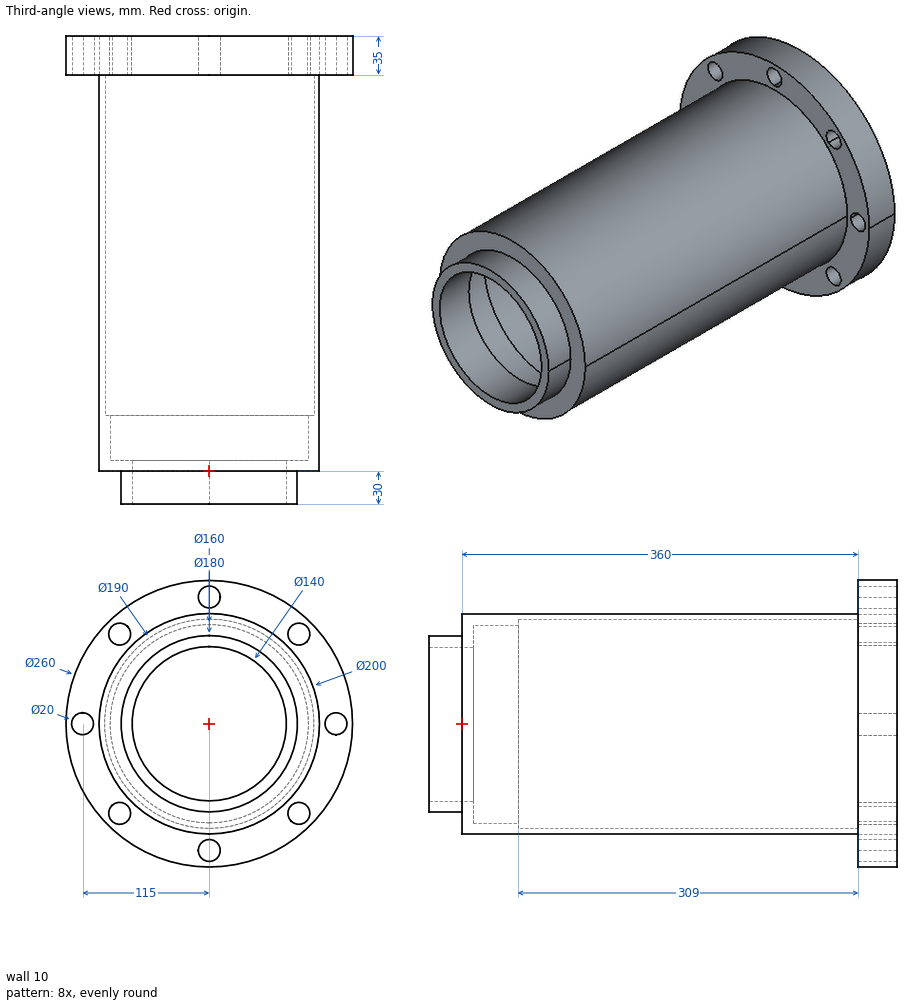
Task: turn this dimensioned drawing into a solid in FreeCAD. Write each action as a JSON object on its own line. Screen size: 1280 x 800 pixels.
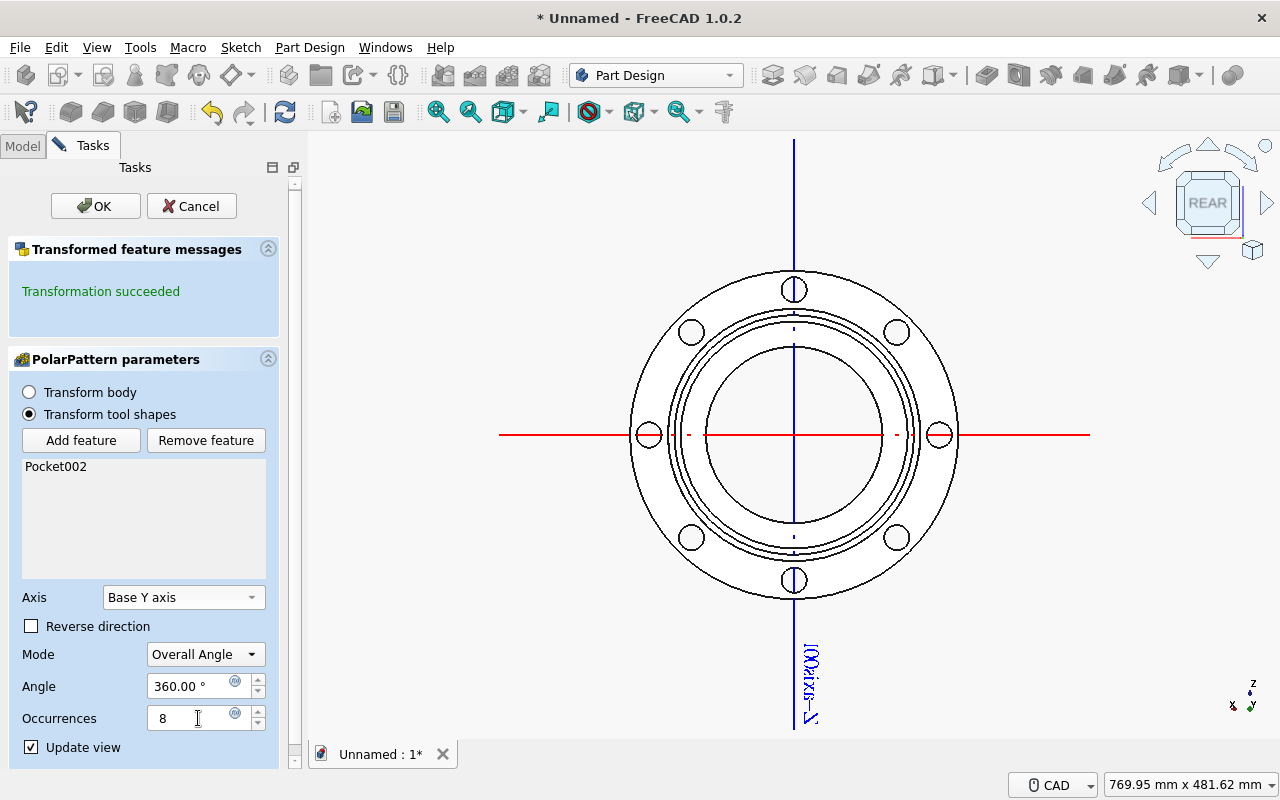
{"action": "left_click", "coordinate": [96, 206]}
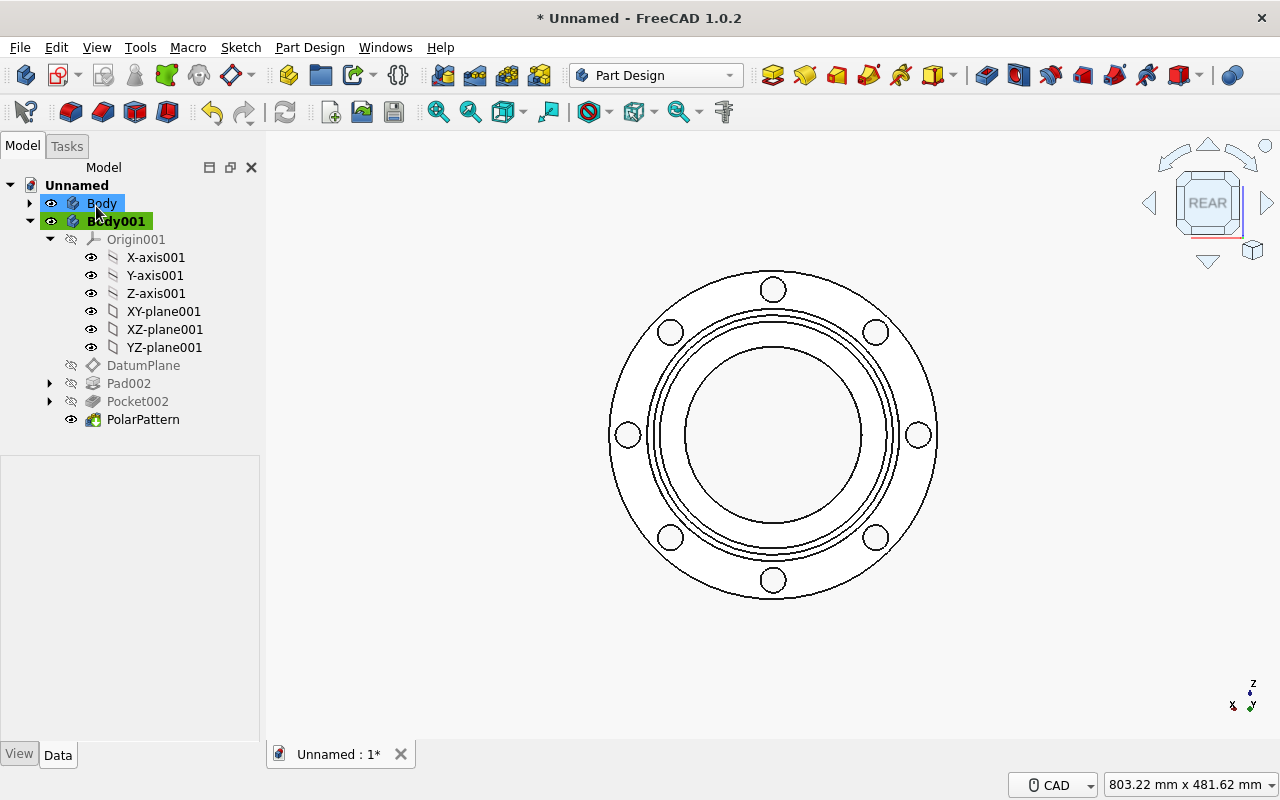
{"action": "key", "text": "0"}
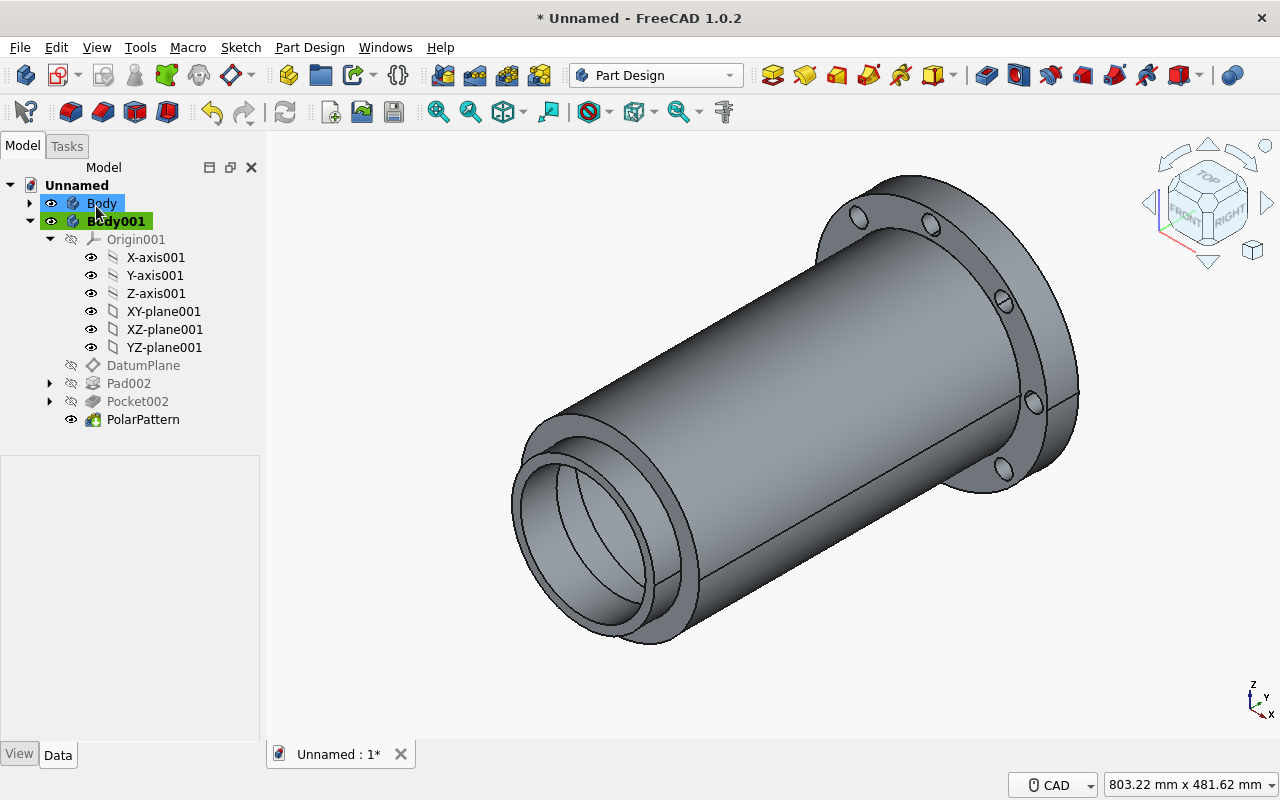
{"action": "left_click", "coordinate": [440, 112]}